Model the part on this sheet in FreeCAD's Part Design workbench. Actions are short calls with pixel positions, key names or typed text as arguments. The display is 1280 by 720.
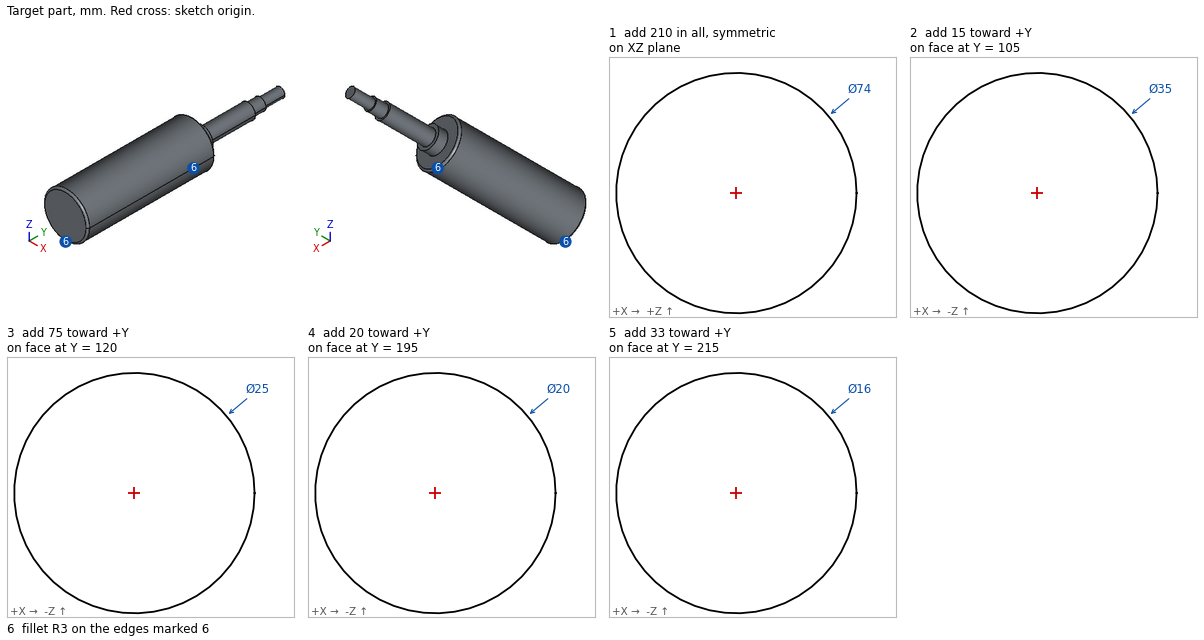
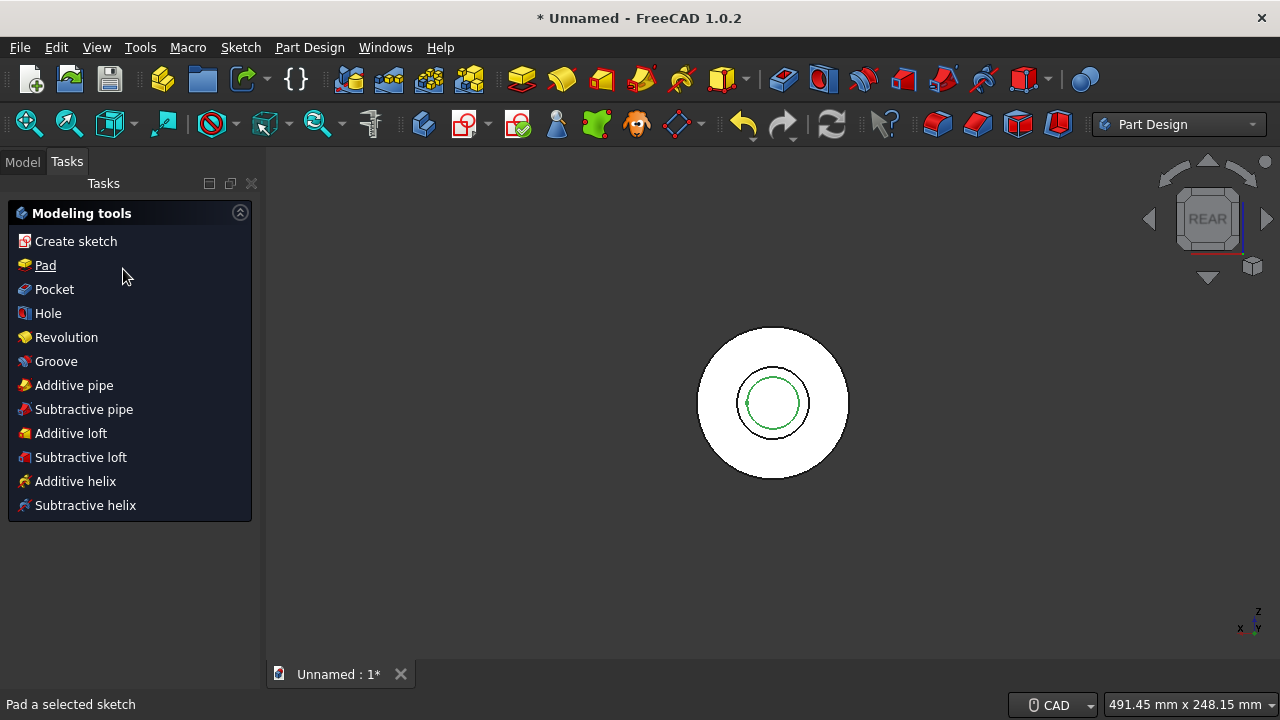
click(522, 80)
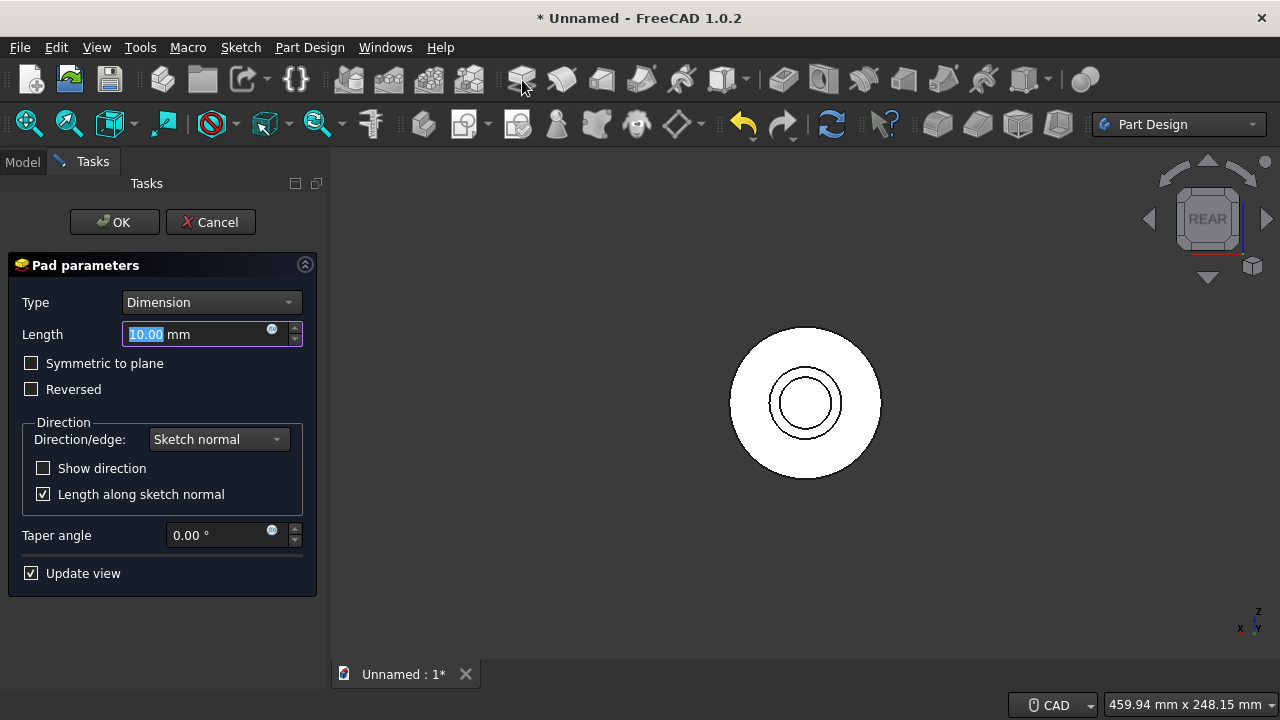
text(75)
key(Tab)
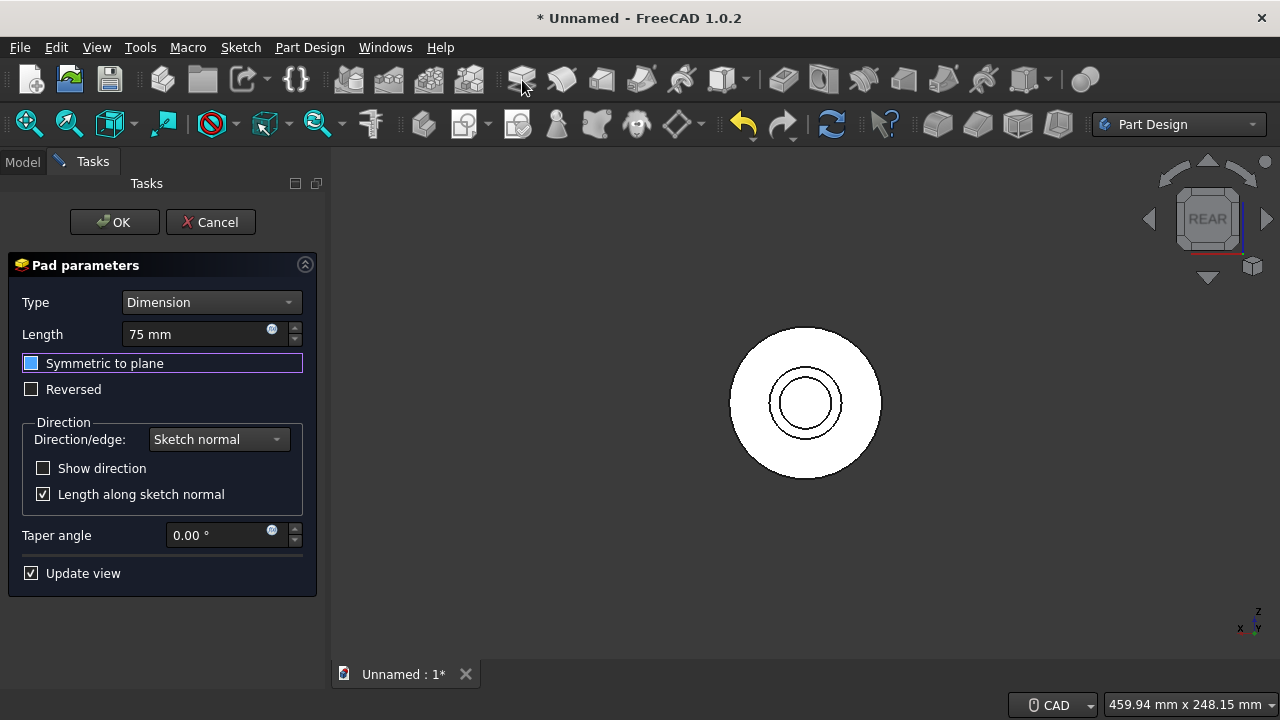
click(115, 222)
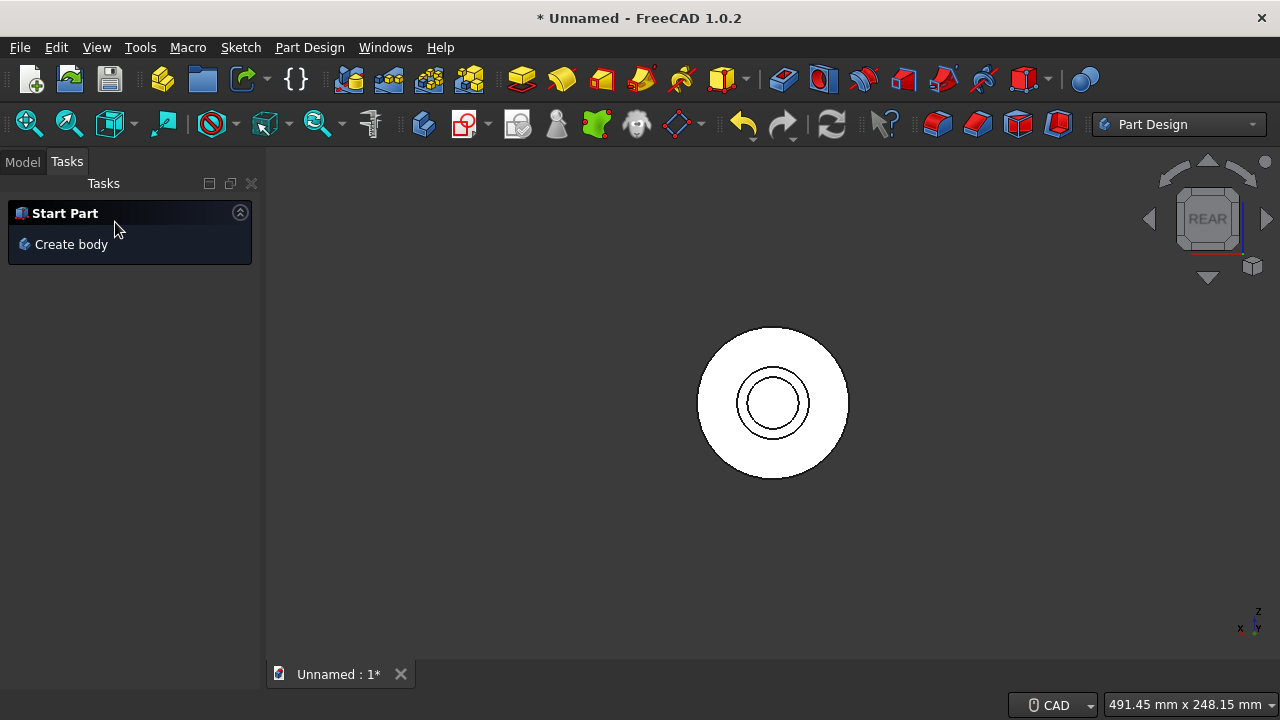
key(v)
key(f)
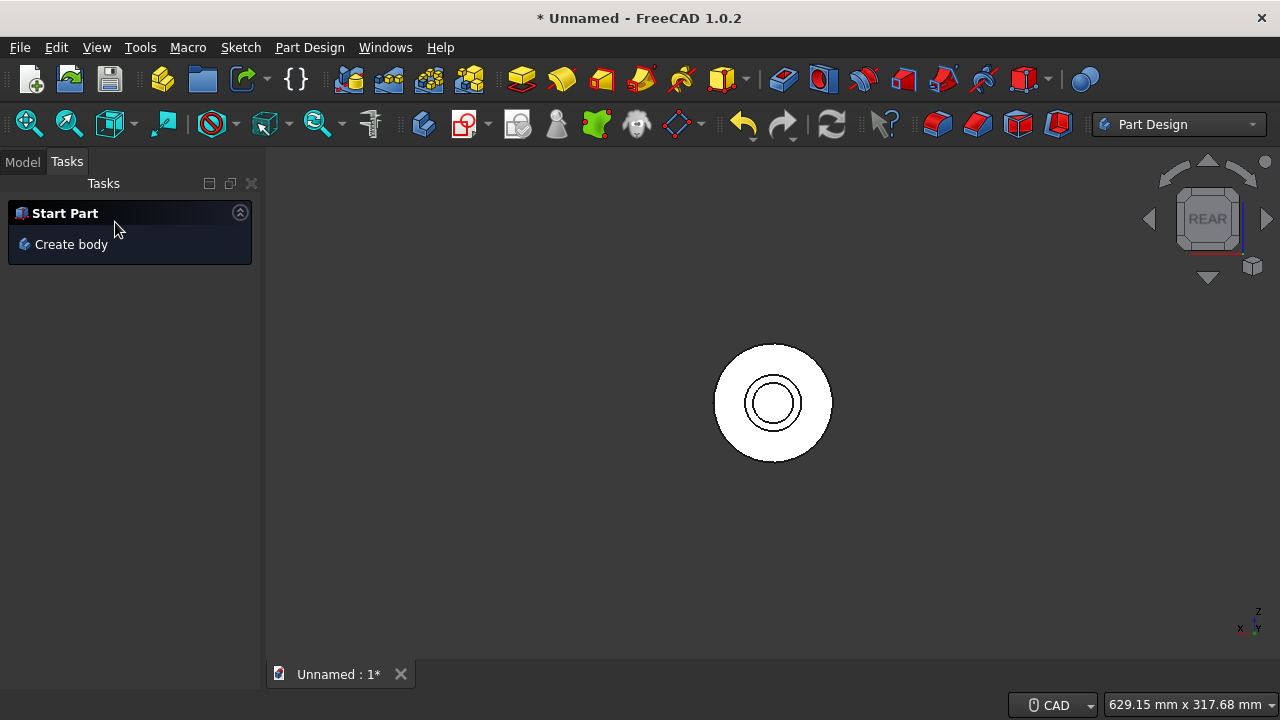
click(773, 402)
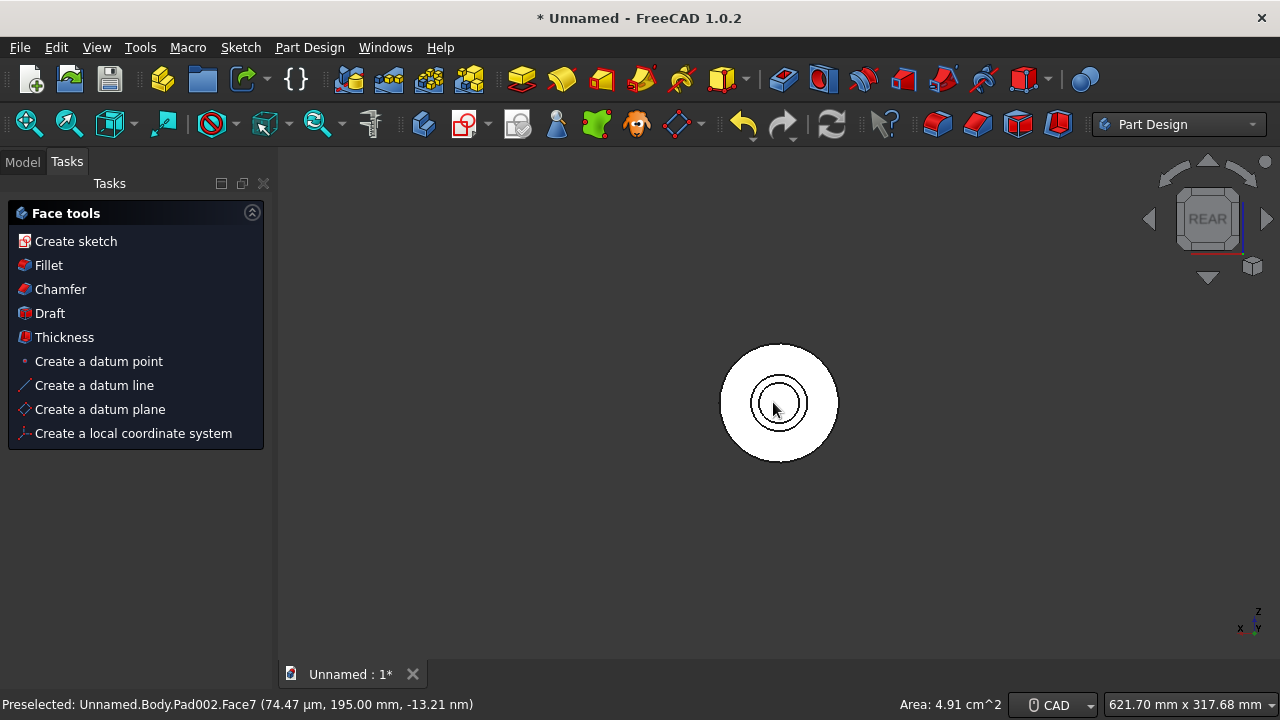
click(464, 124)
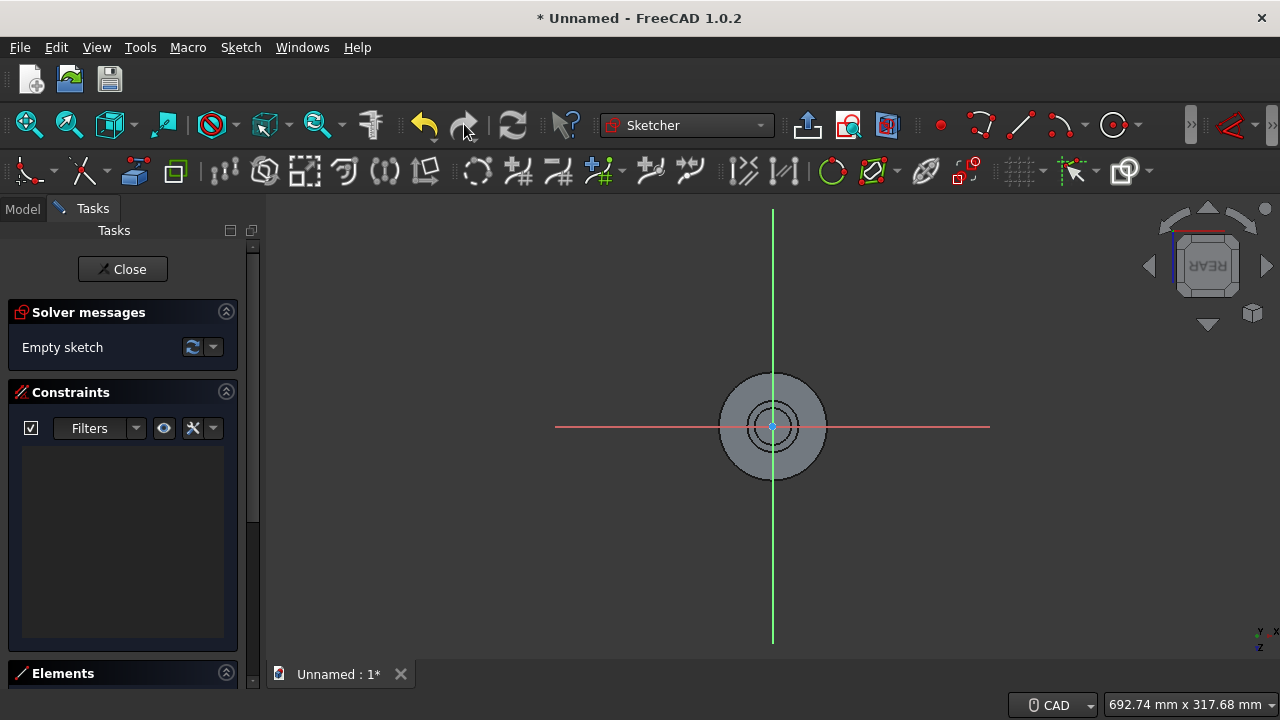
scroll(781, 426, up, 11)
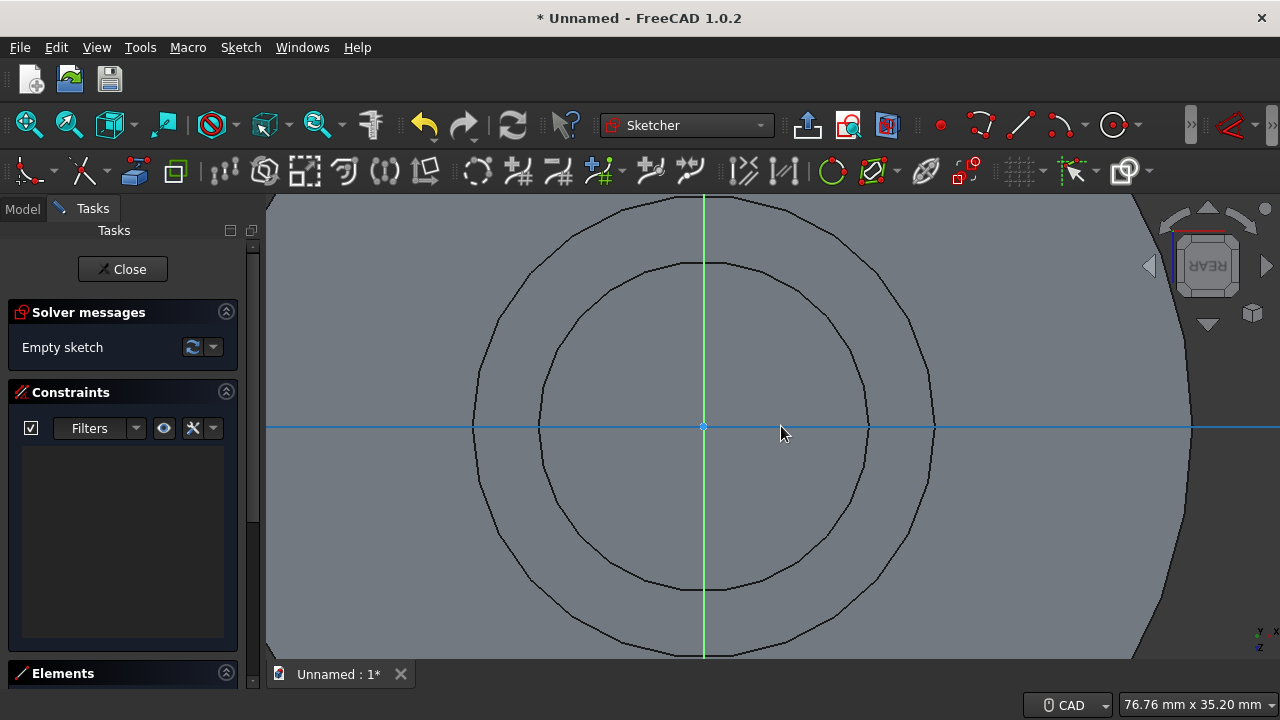
click(1114, 126)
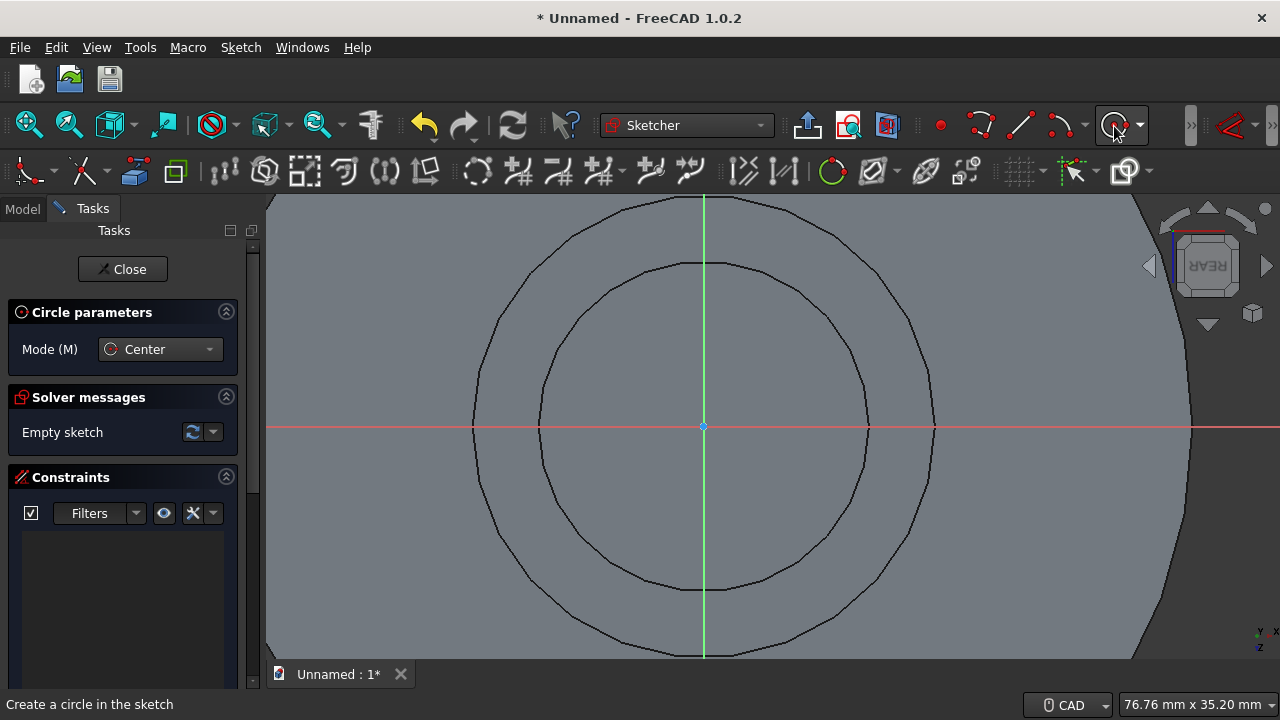
click(704, 426)
move(797, 333)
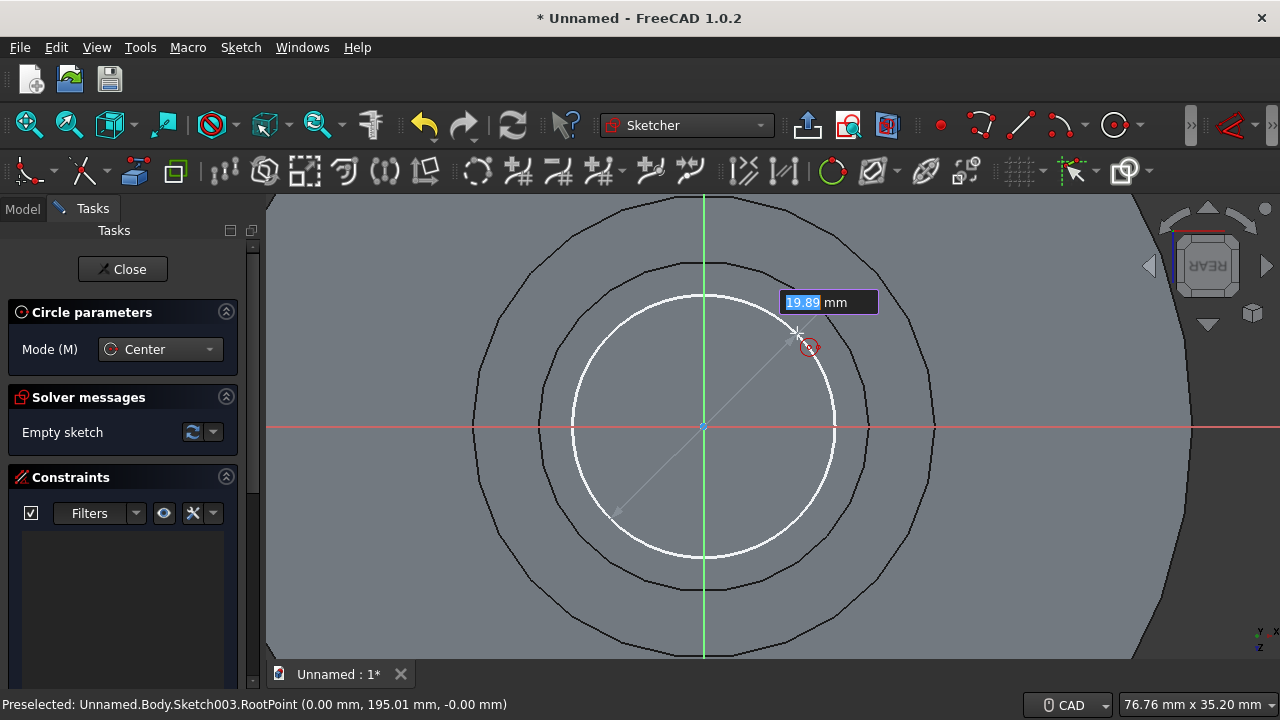
text(20)
key(Return)
key(Escape)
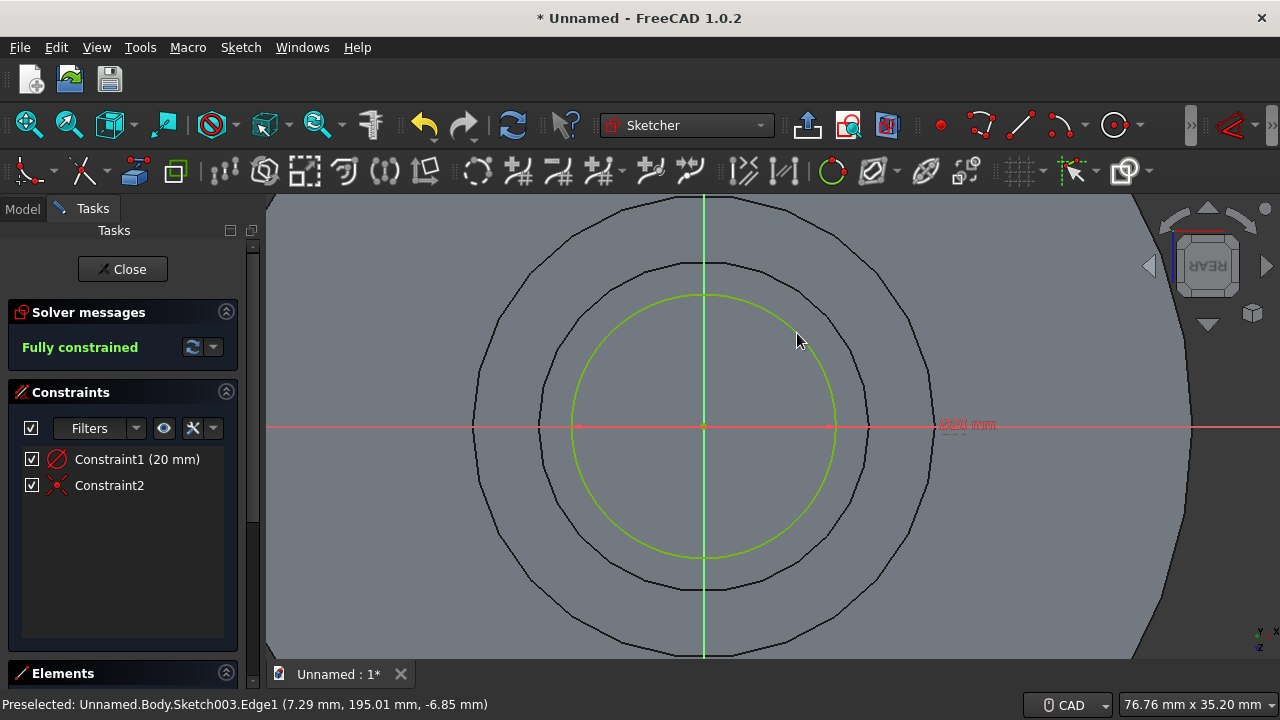
click(123, 269)